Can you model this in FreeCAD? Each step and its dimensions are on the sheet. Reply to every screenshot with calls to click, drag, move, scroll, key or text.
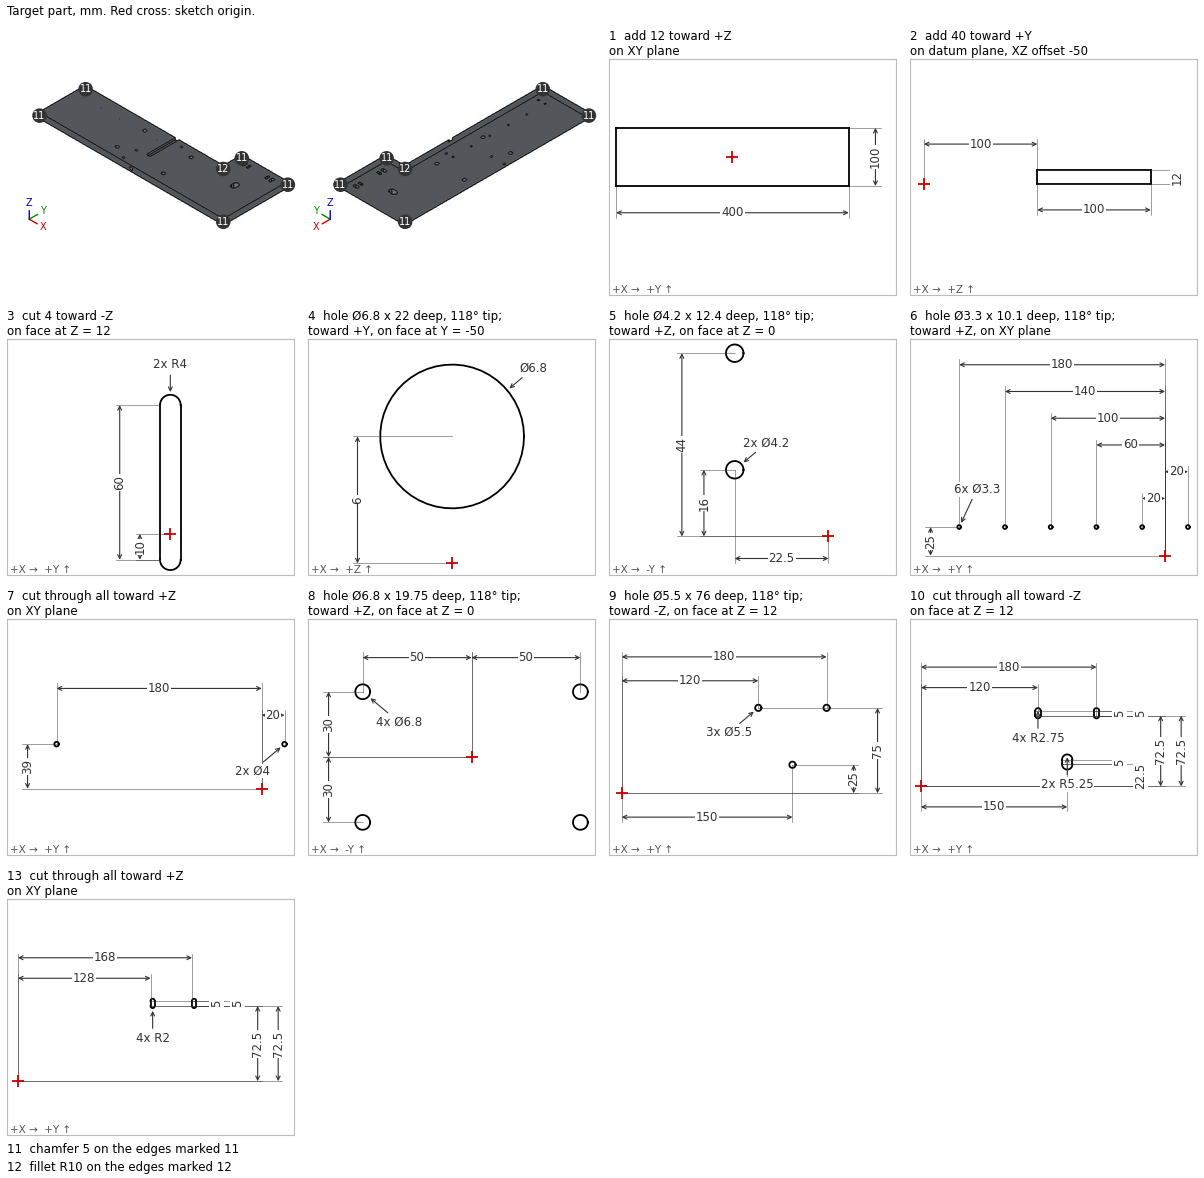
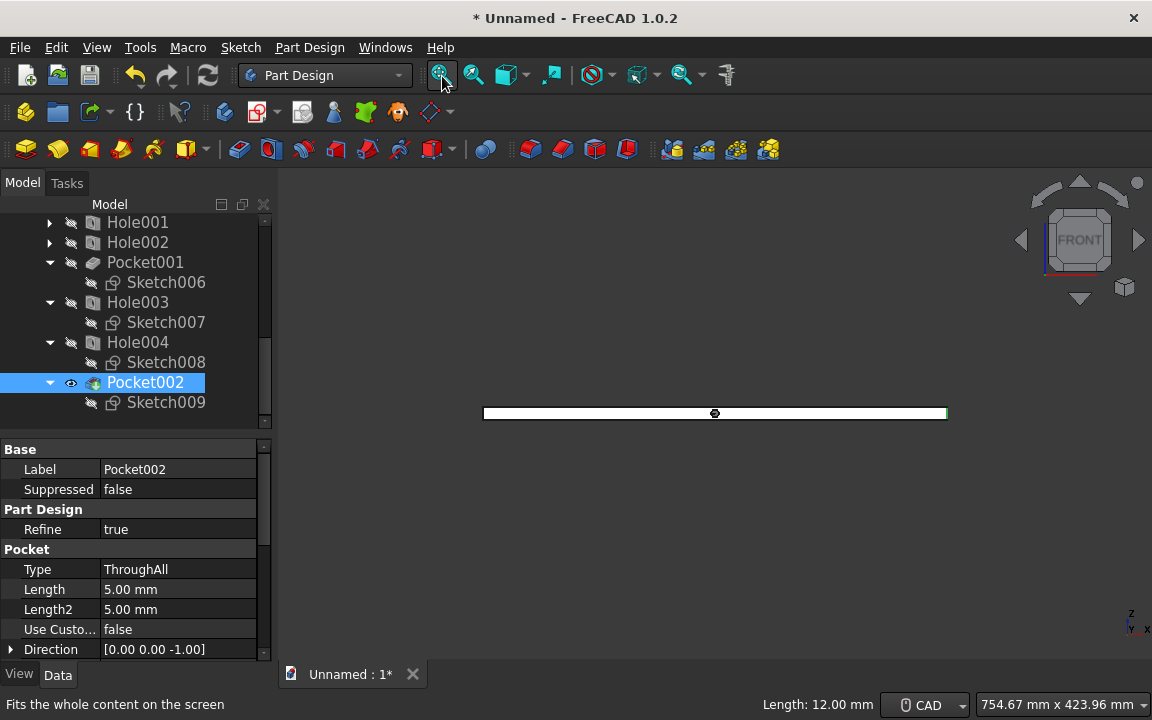
click(483, 412, ctrl)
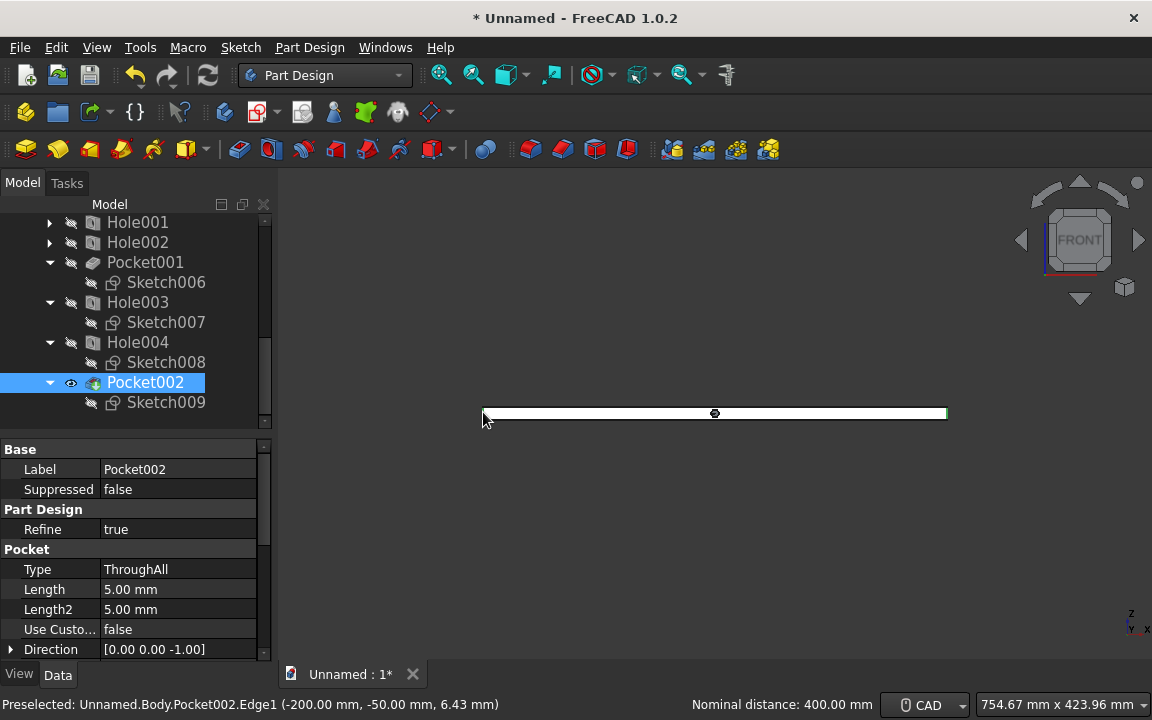
scroll(831, 412, up, 6)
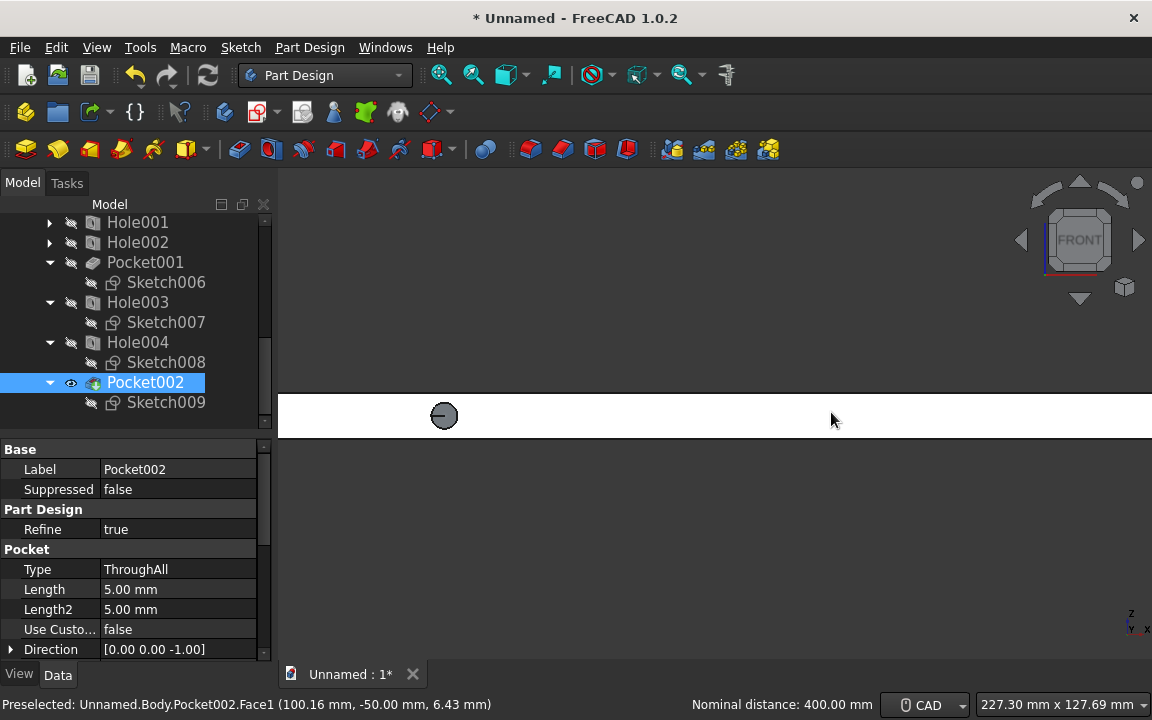
click(442, 76)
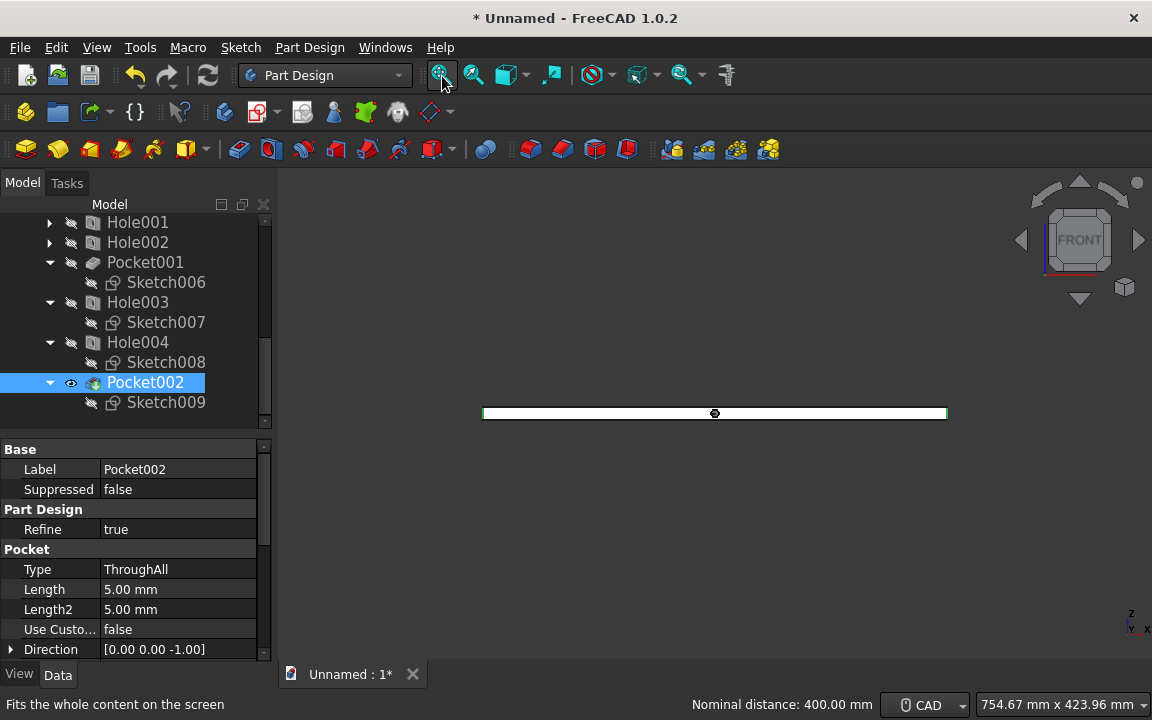
key(3)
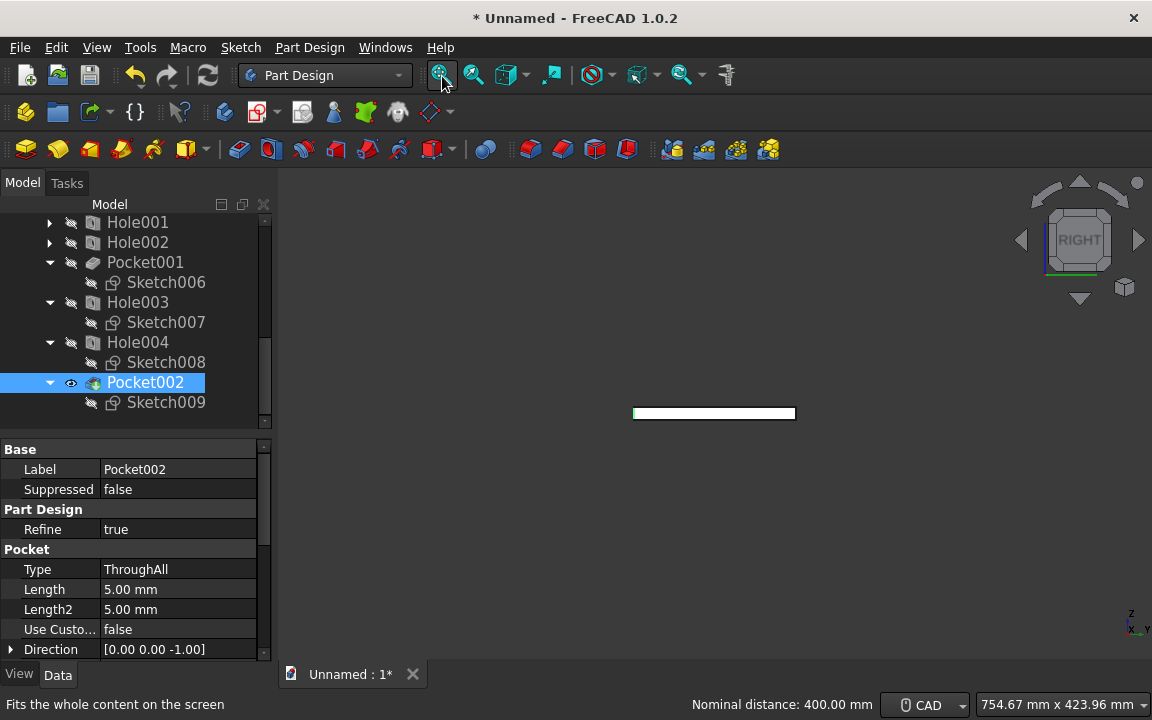
click(442, 76)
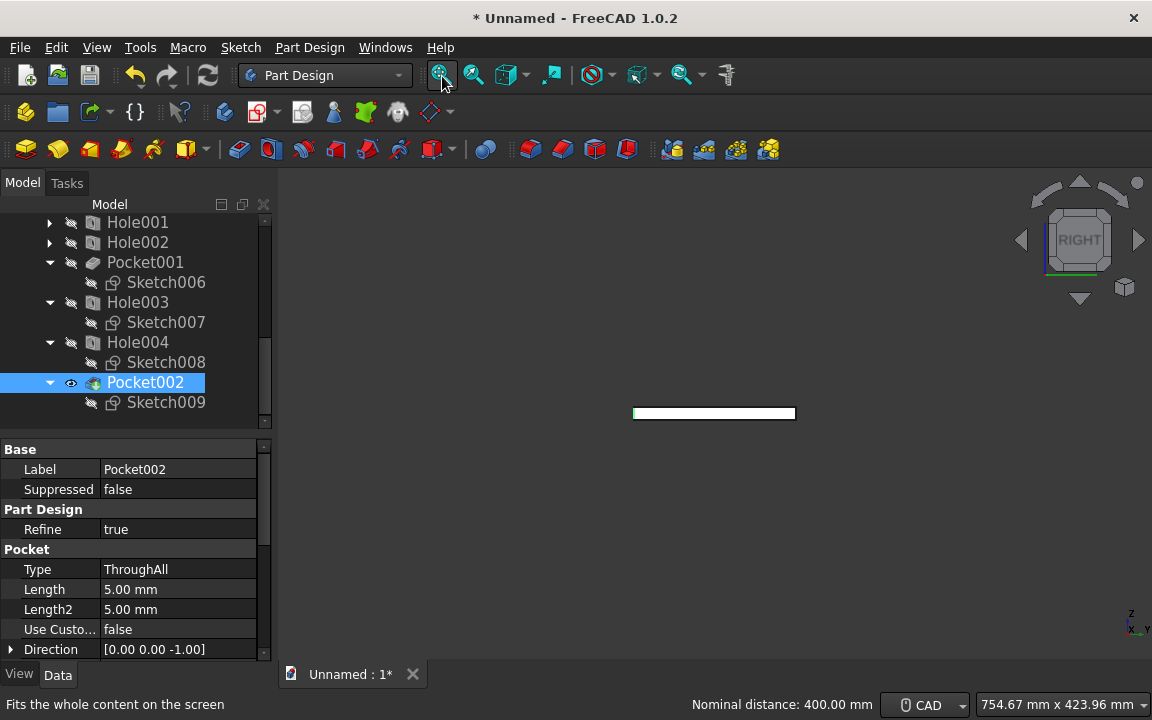
click(796, 412, ctrl)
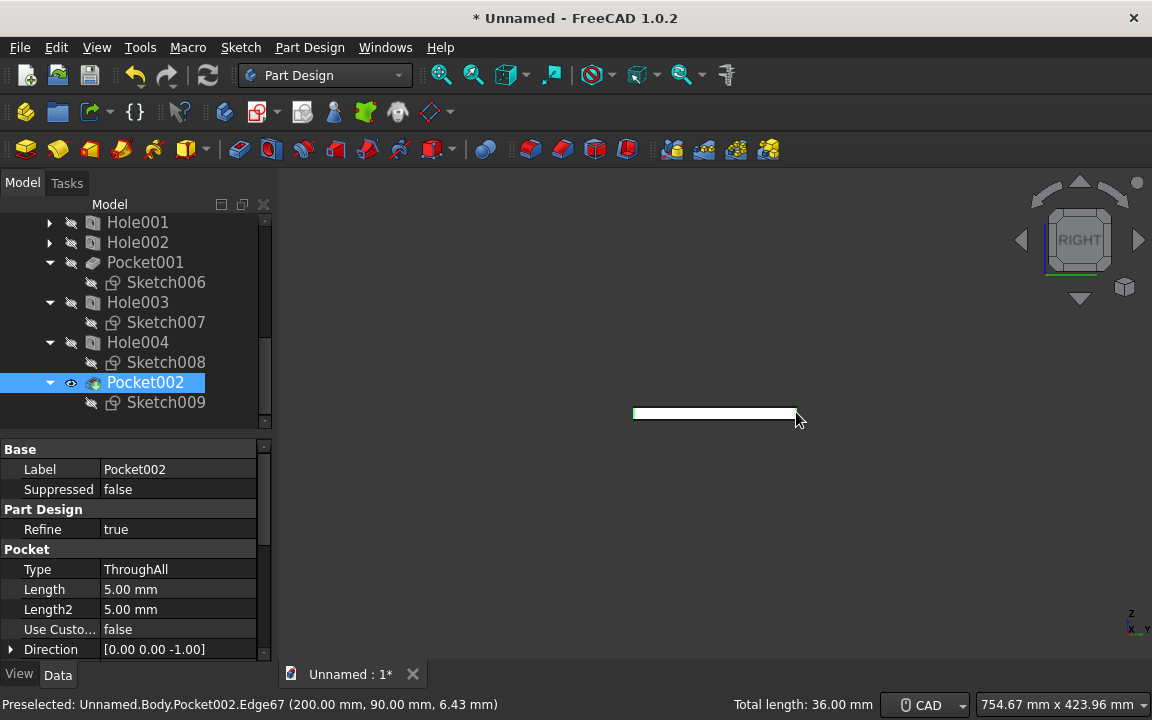
scroll(796, 412, up, 6)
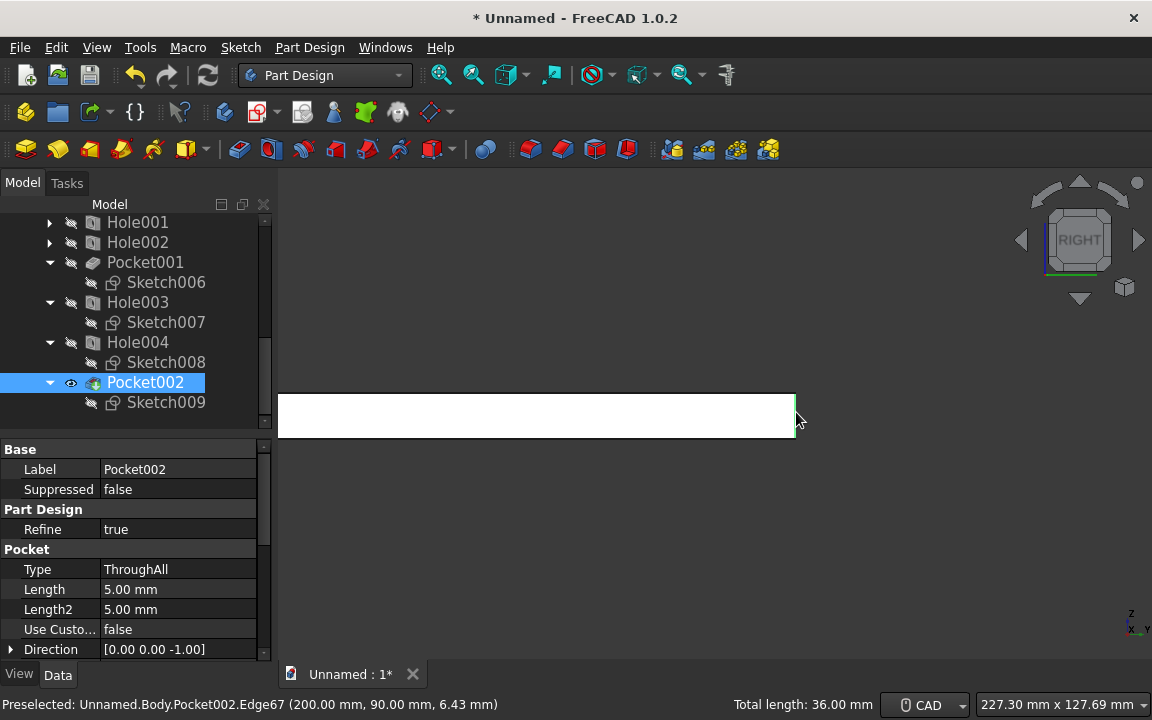
click(442, 76)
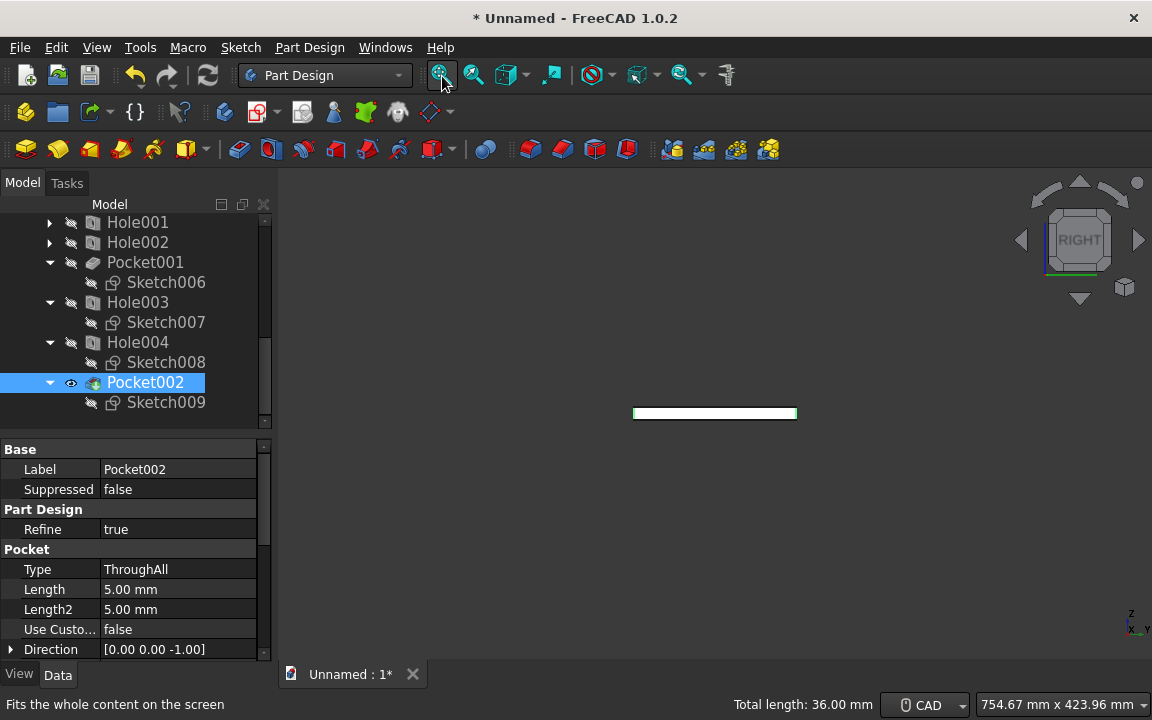
key(5)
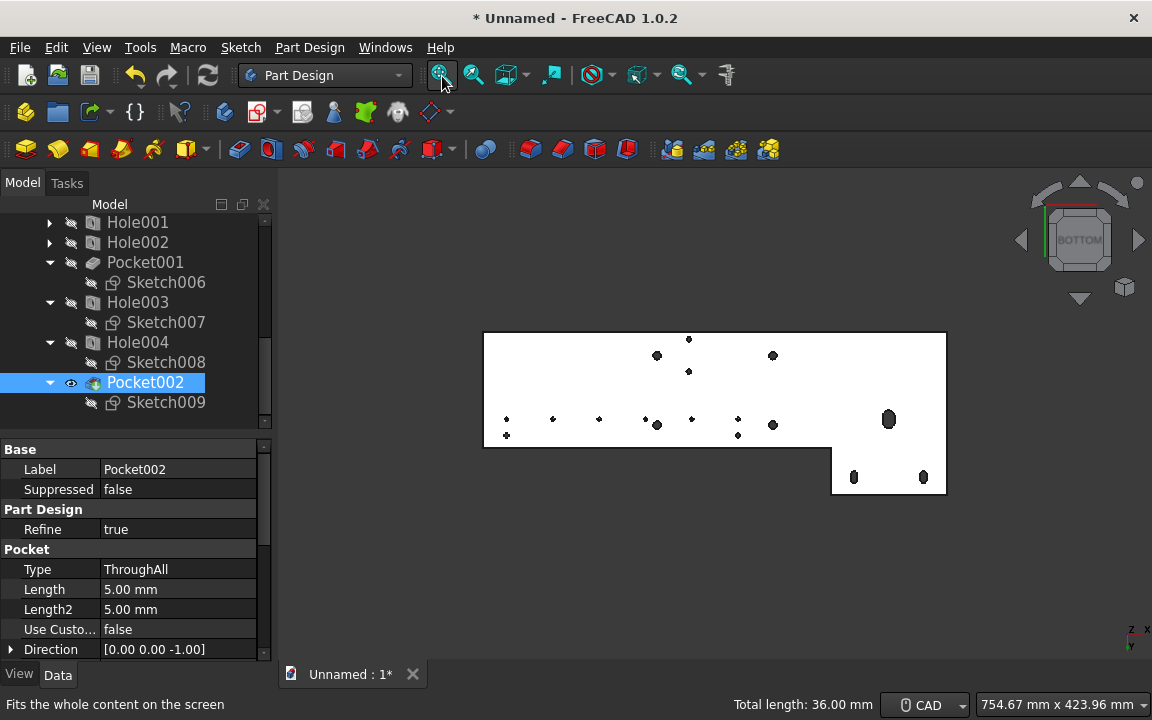
scroll(831, 494, up, 6)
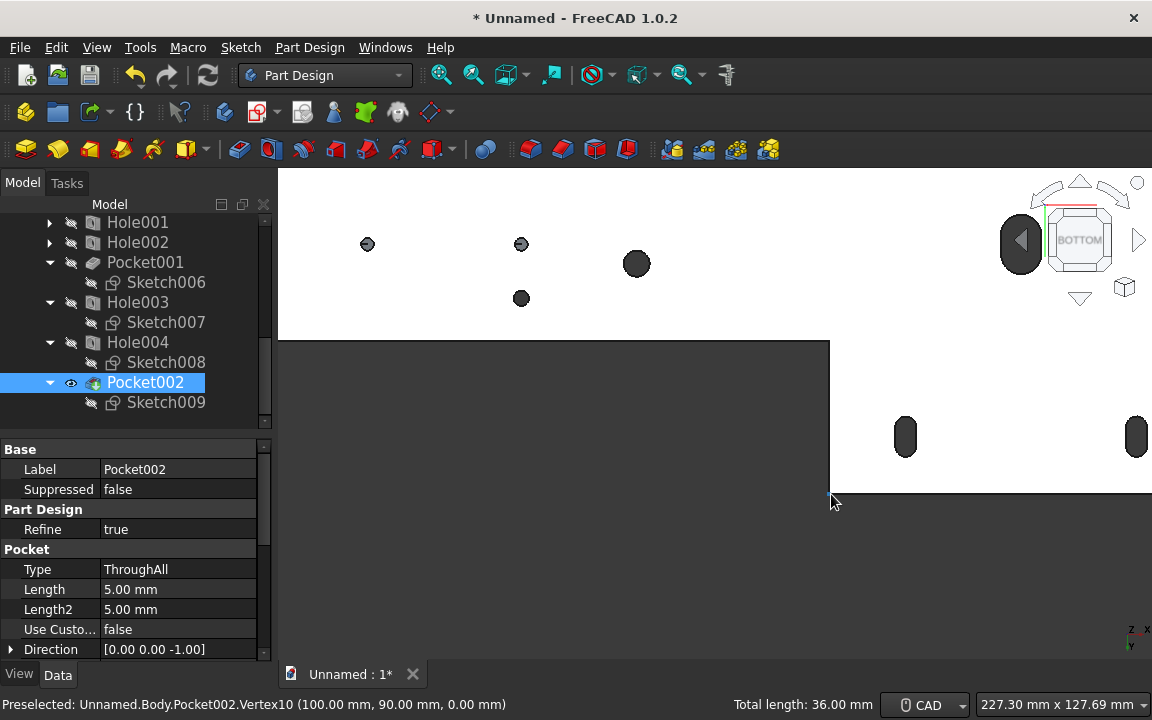
click(442, 76)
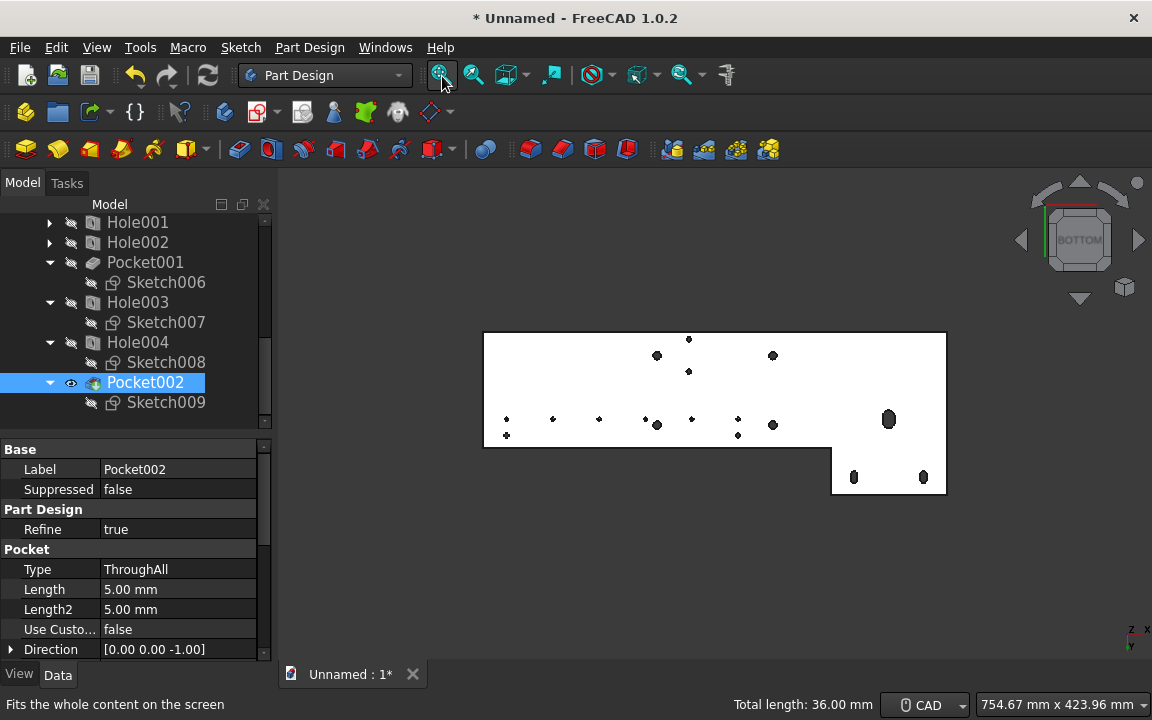
key(4)